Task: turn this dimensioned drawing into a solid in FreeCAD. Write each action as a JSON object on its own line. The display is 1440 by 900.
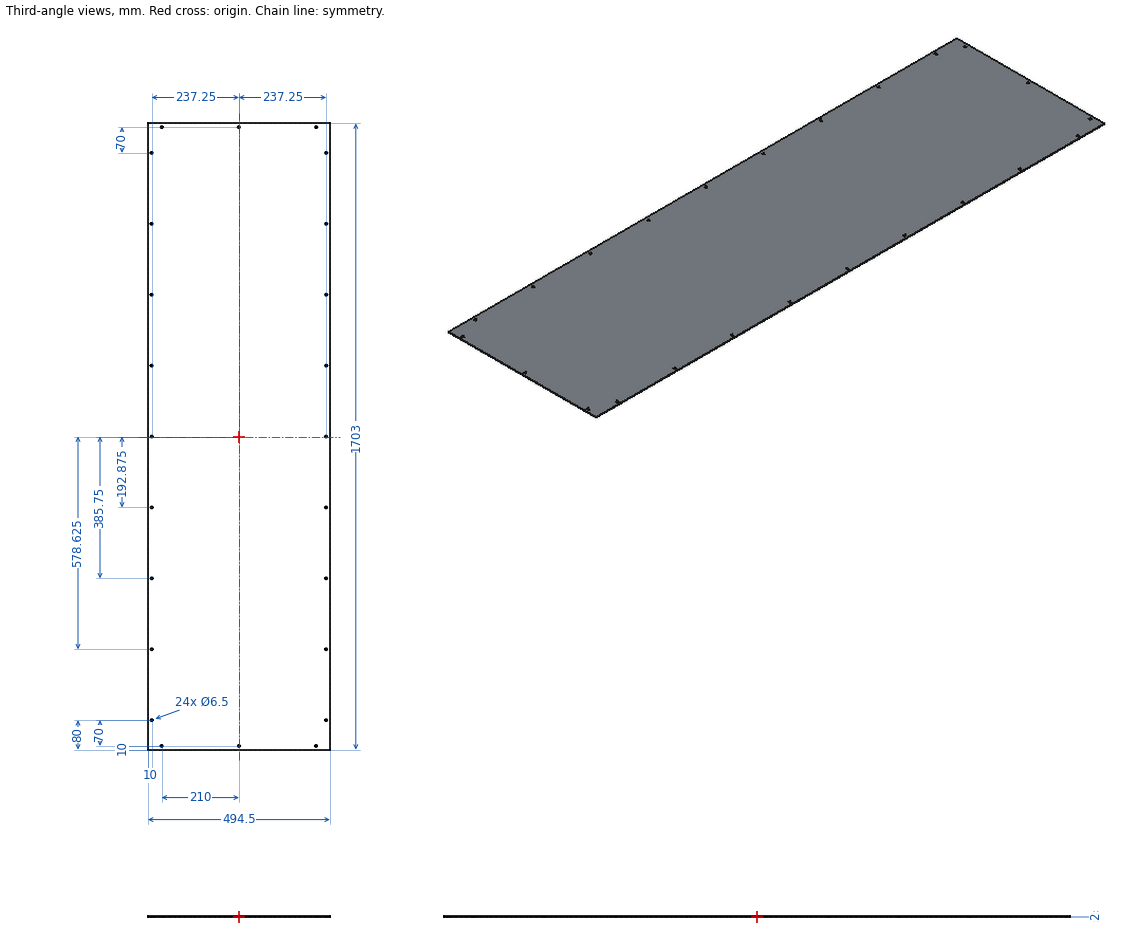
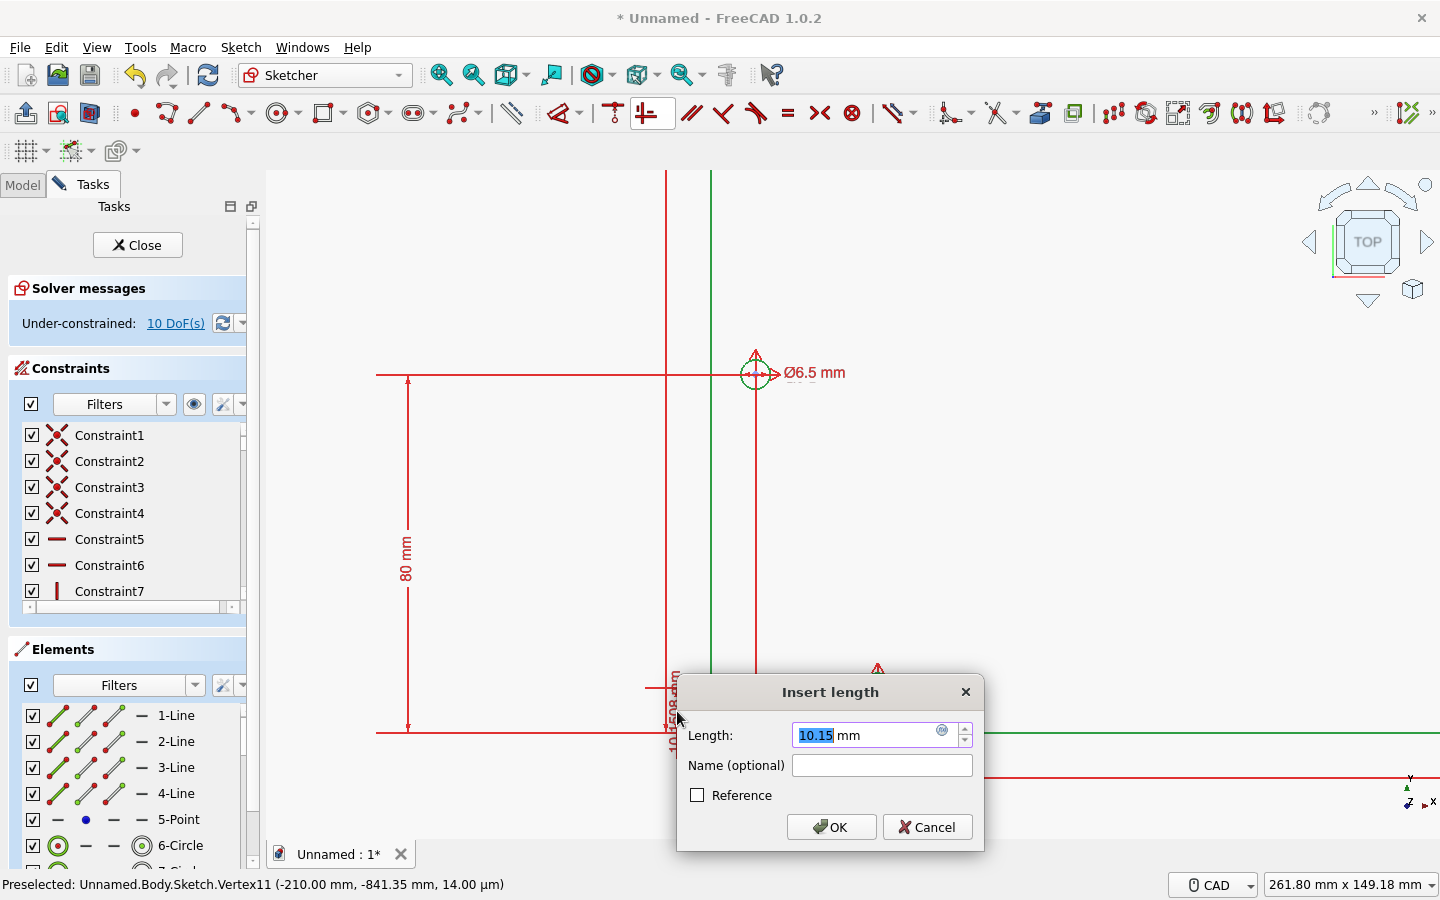
{"action": "type", "text": "10"}
{"action": "key", "text": "Return"}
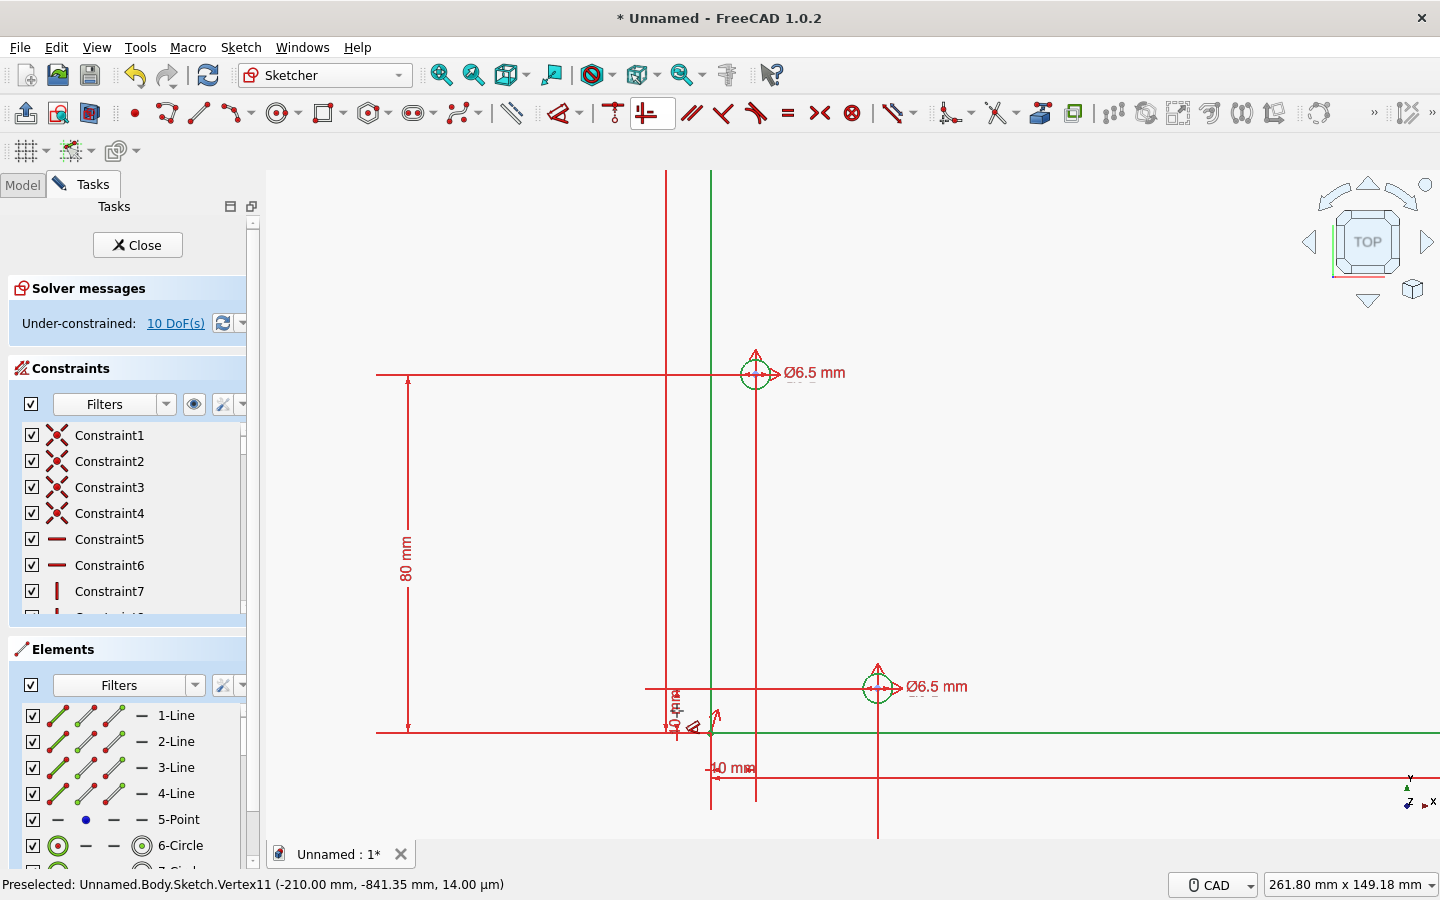
{"action": "left_click", "coordinate": [711, 733]}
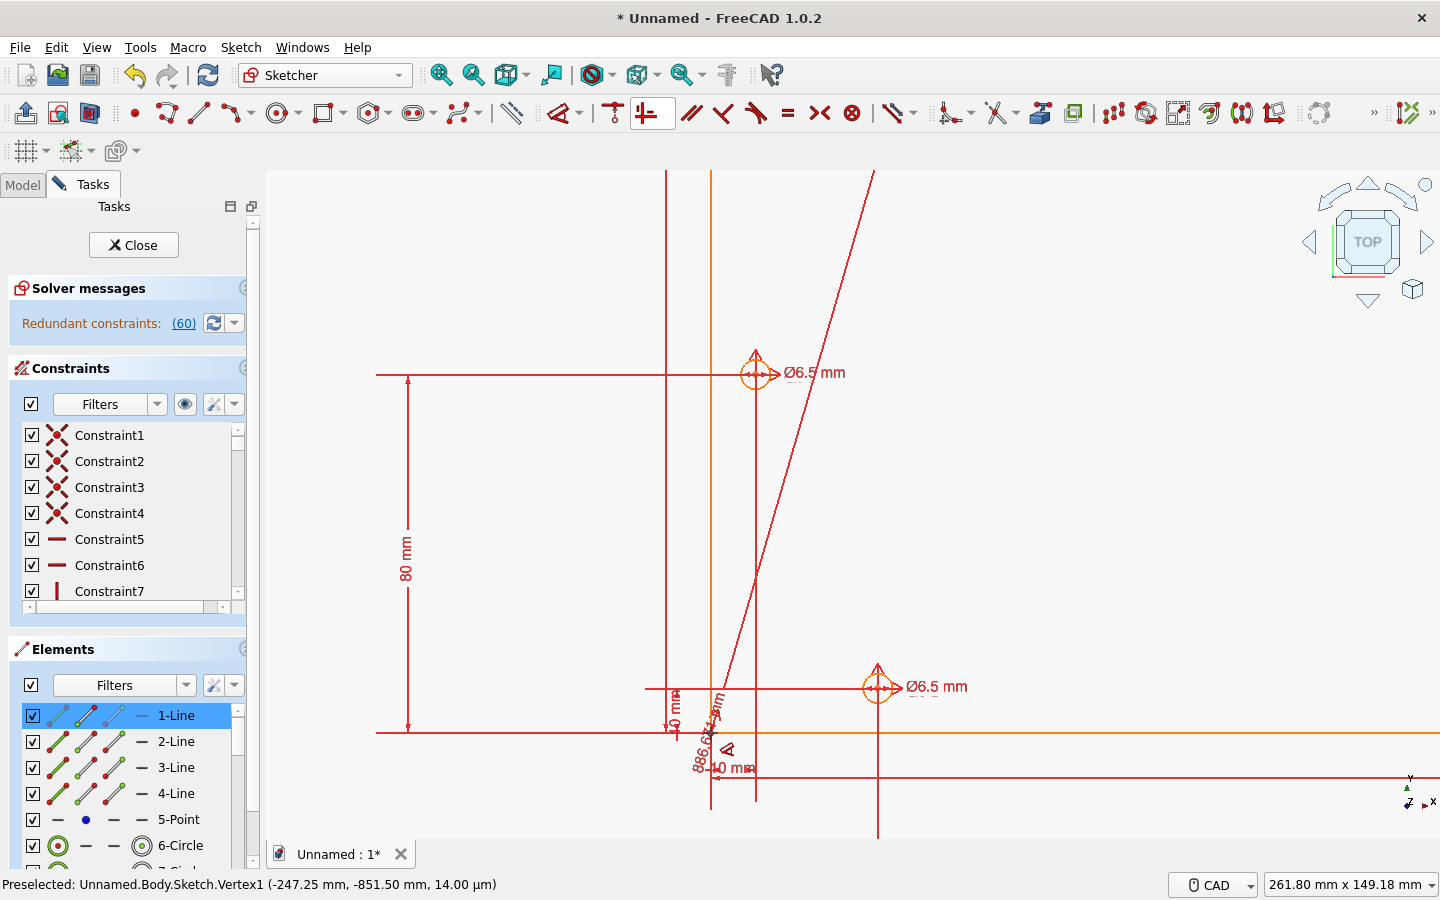
{"action": "scroll", "coordinate": [717, 737], "scroll_direction": "down", "scroll_amount": 14}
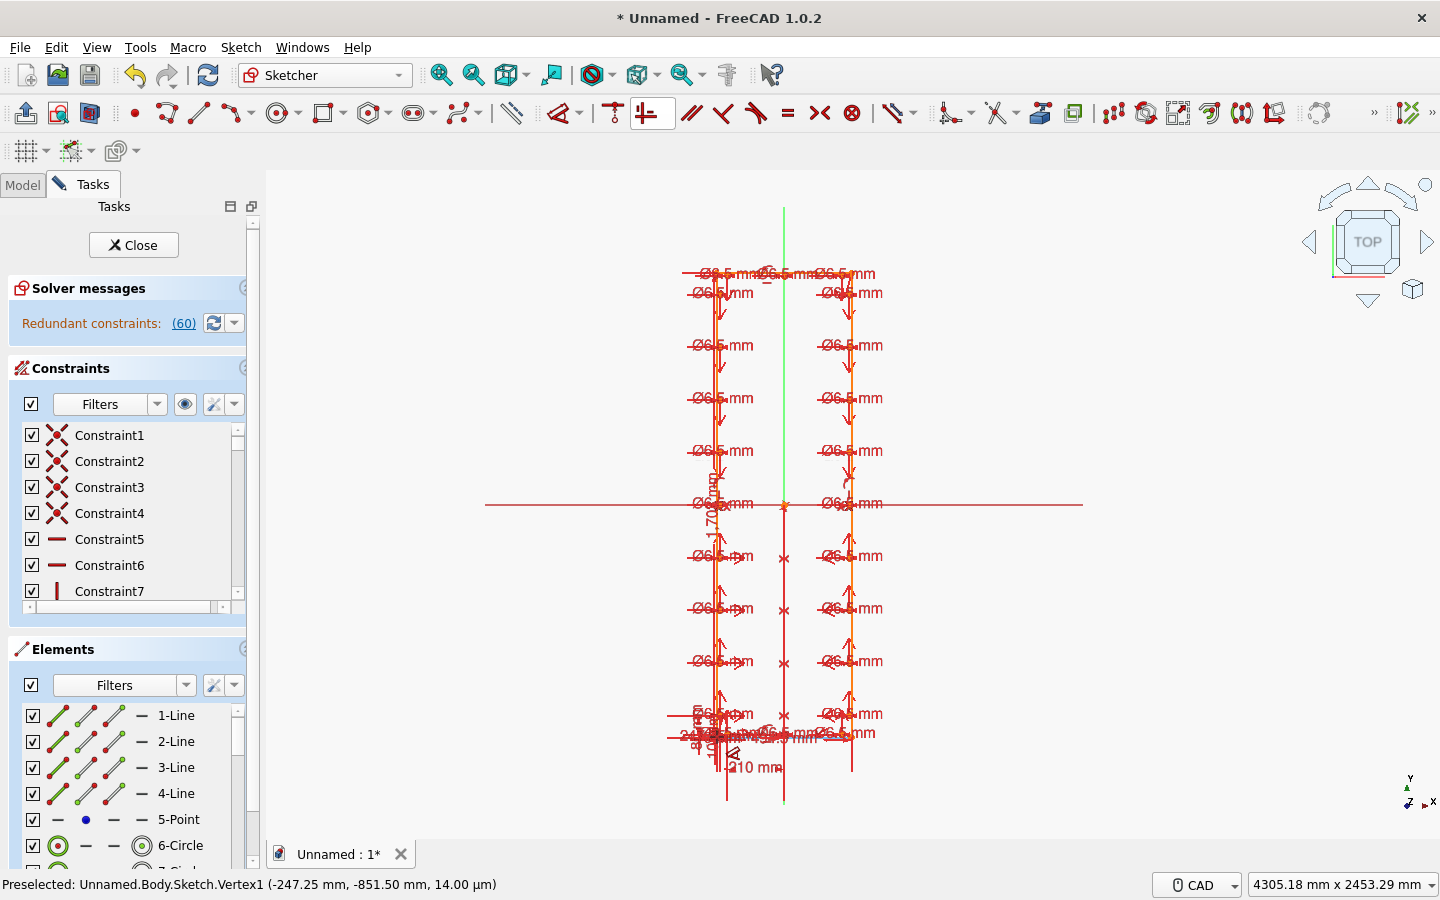
{"action": "scroll", "coordinate": [720, 663], "scroll_direction": "up", "scroll_amount": 14}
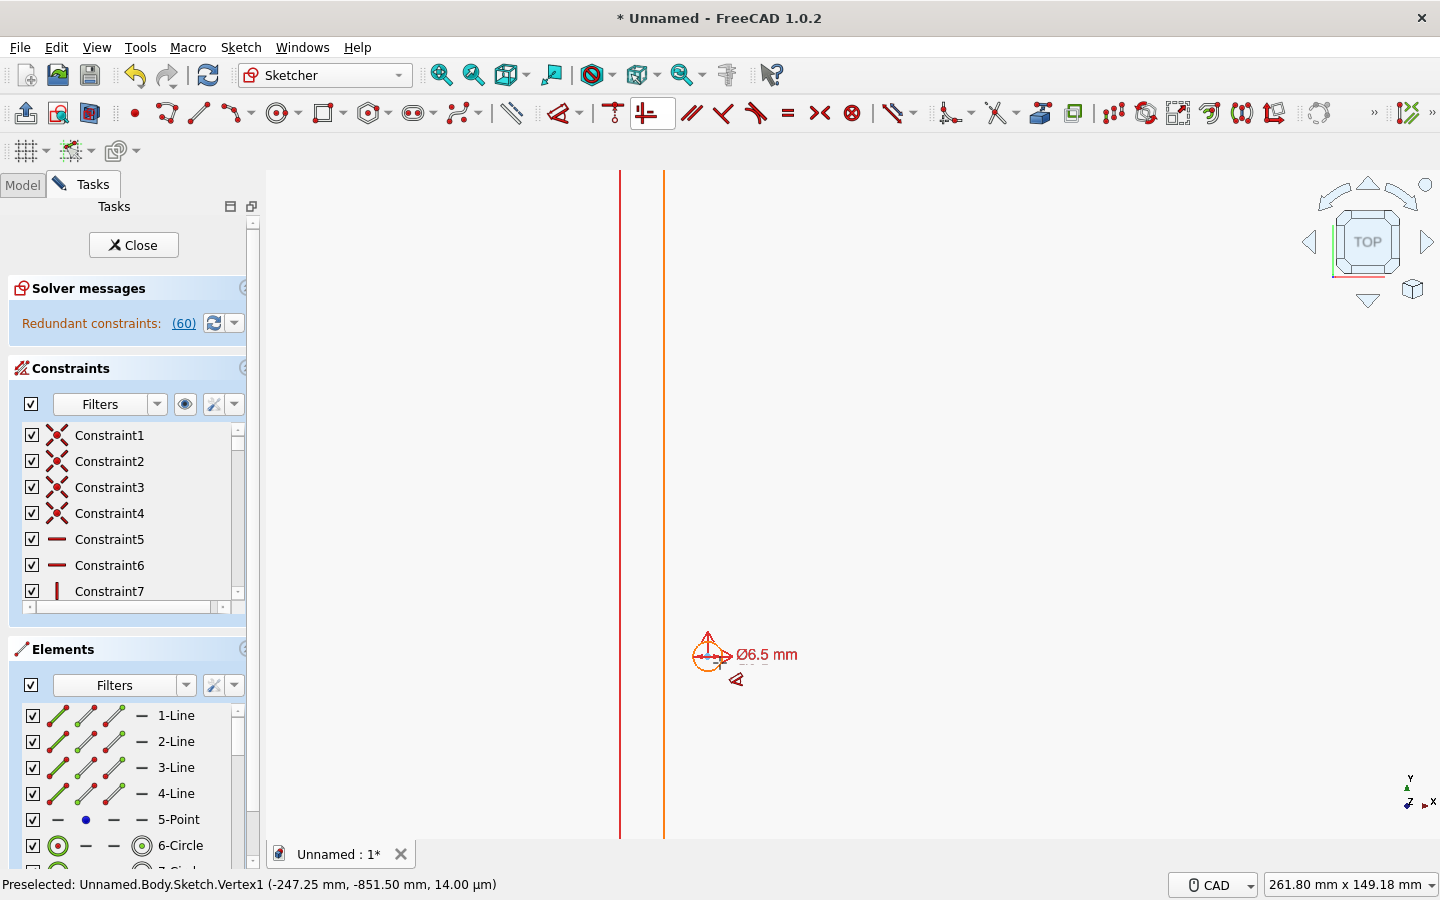
{"action": "left_click", "coordinate": [708, 657]}
{"action": "left_click", "coordinate": [686, 623]}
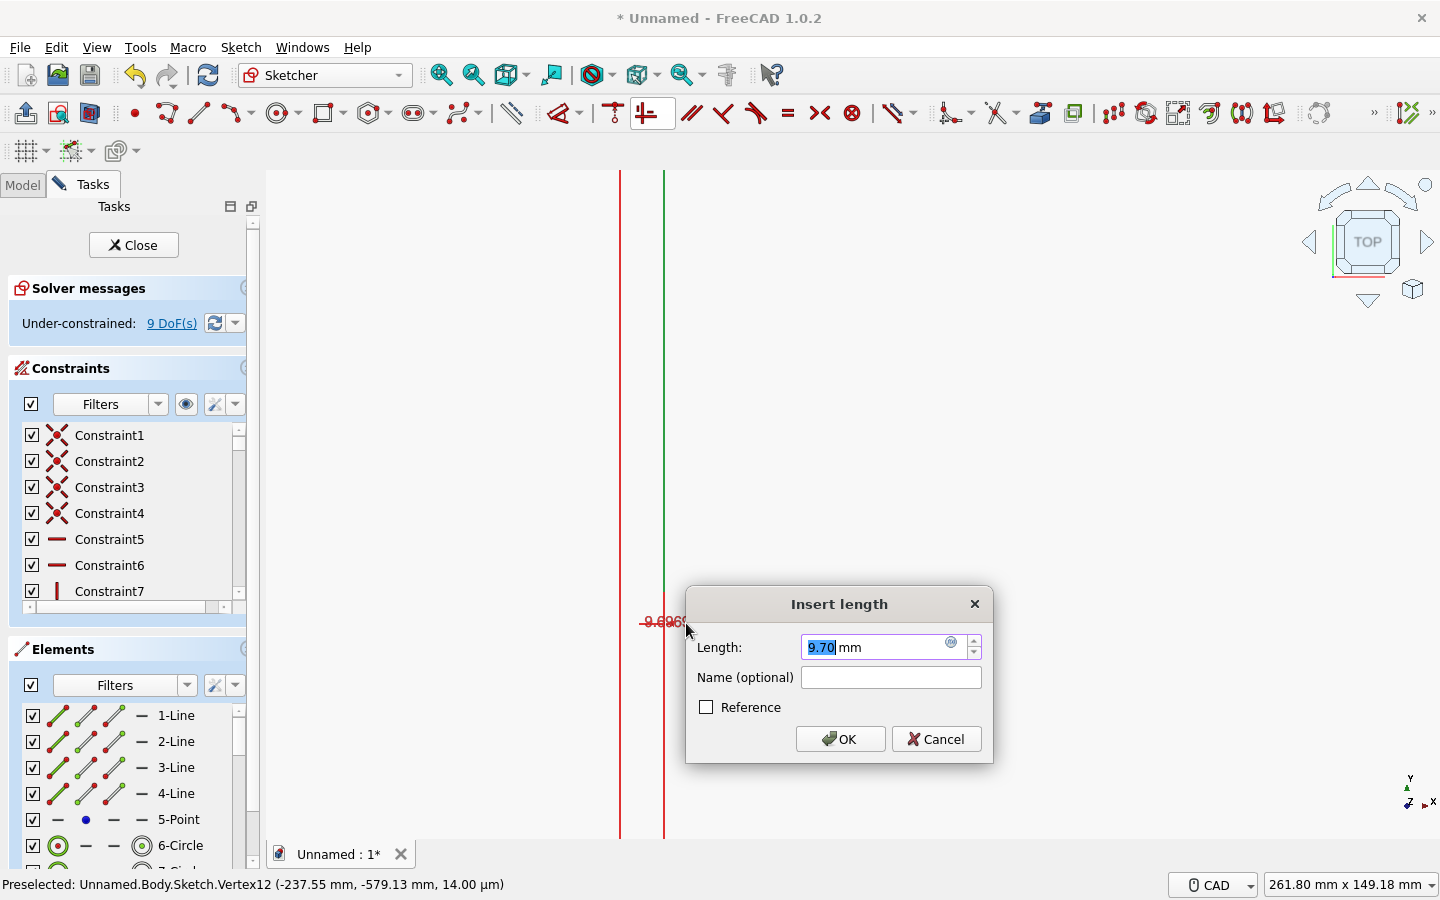
{"action": "type", "text": "10"}
{"action": "key", "text": "Return"}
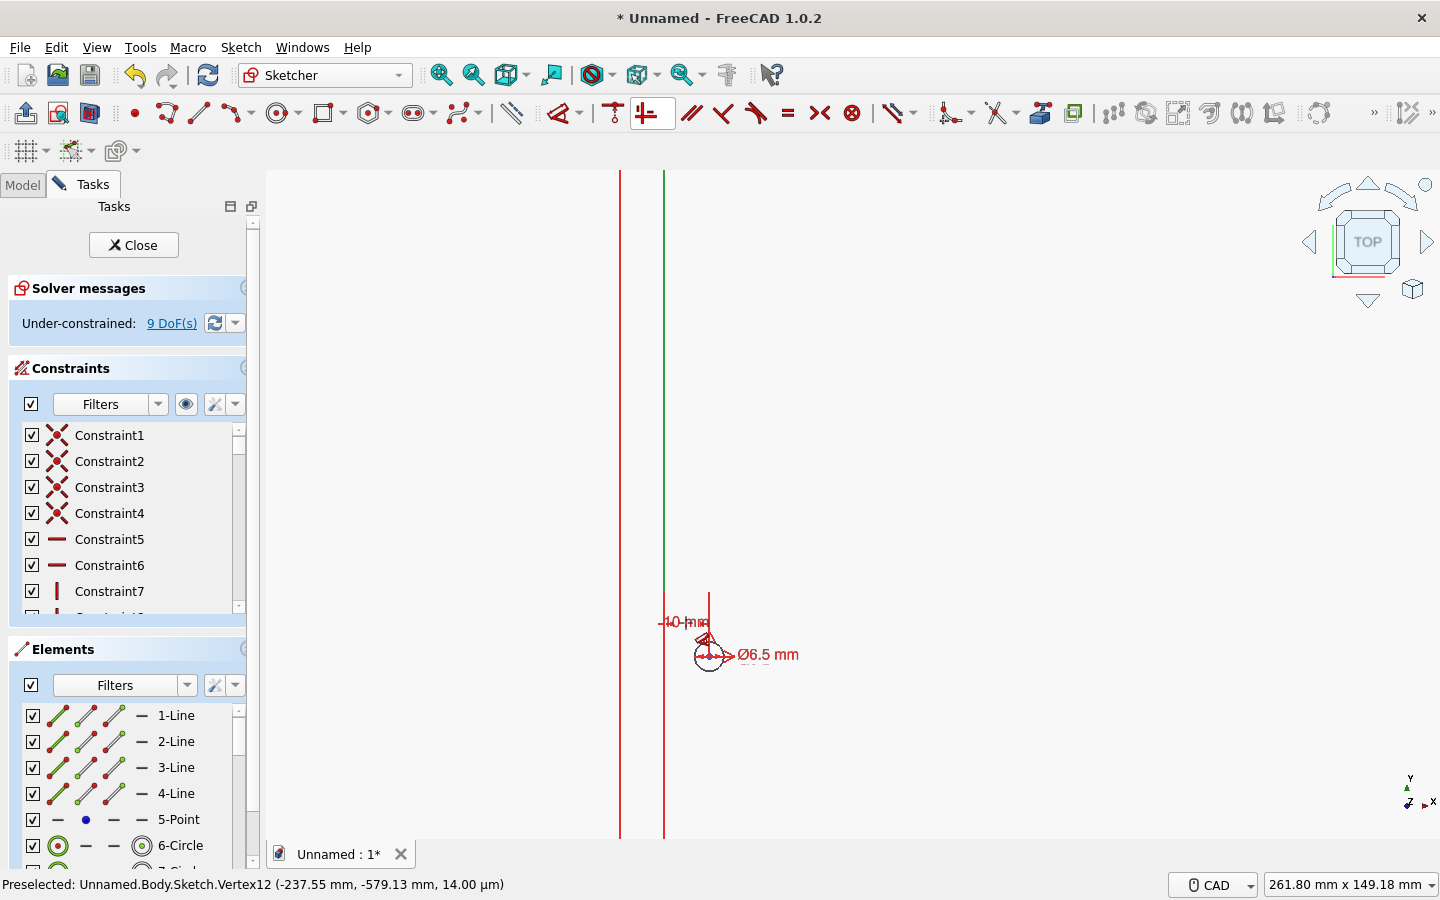
{"action": "scroll", "coordinate": [720, 663], "scroll_direction": "down", "scroll_amount": 14}